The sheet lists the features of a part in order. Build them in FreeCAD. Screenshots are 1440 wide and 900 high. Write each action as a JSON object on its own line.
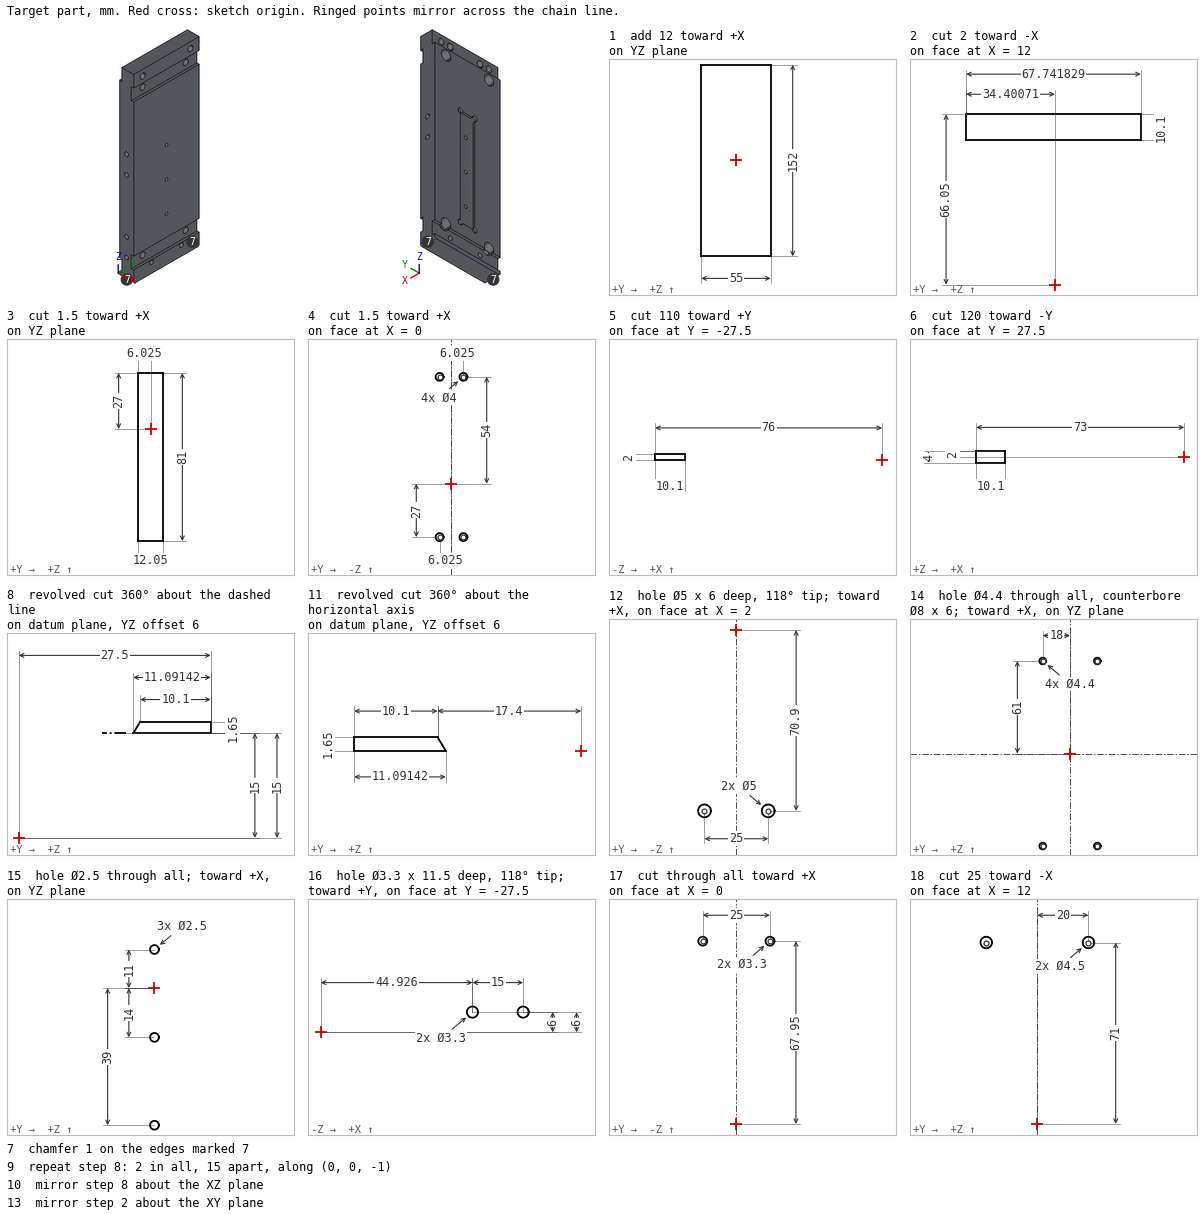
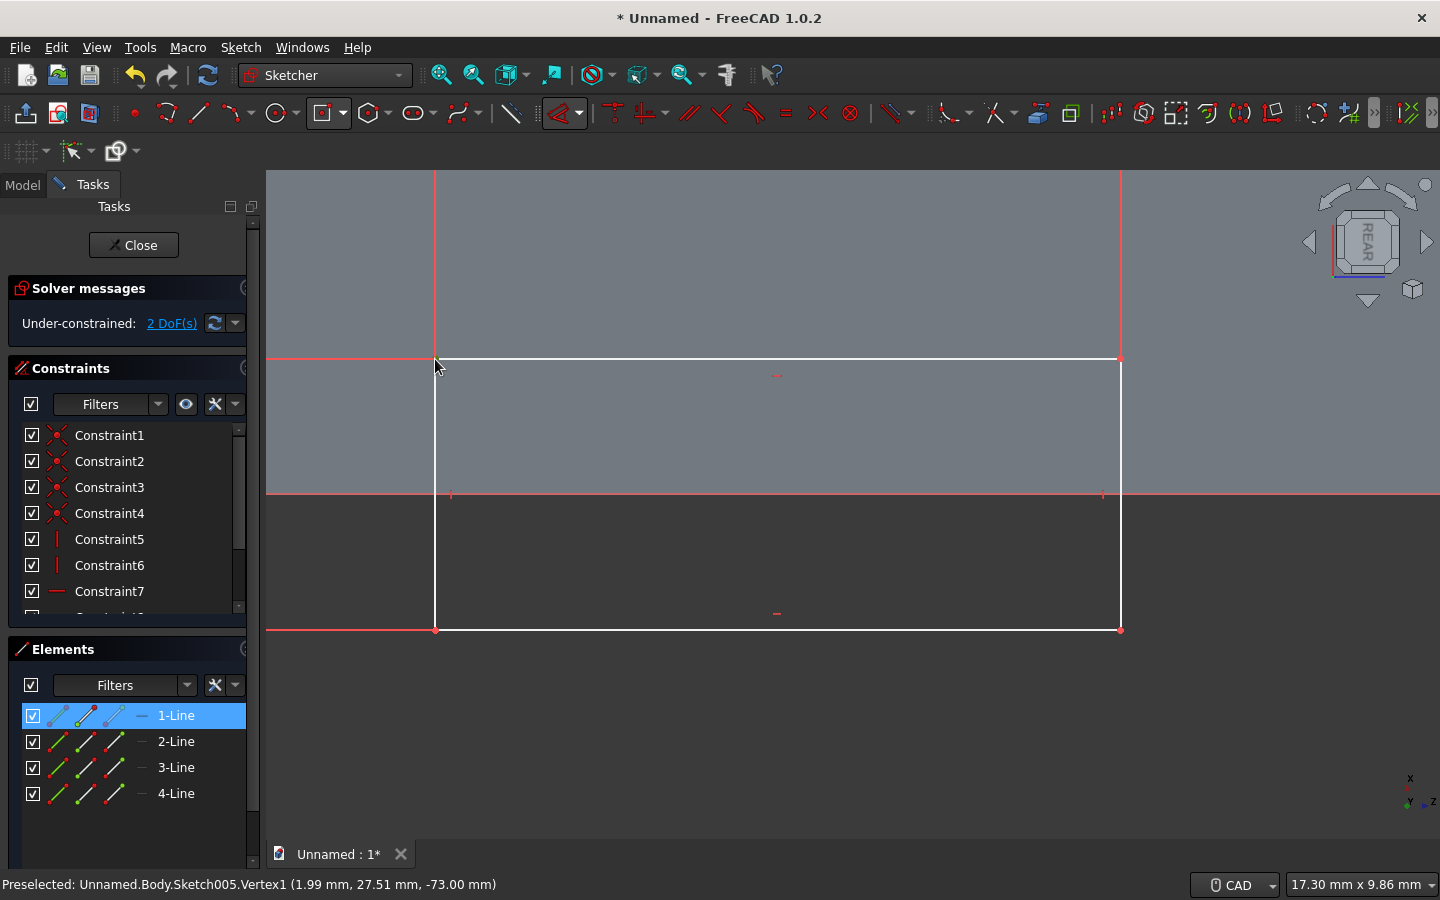
{"action": "left_click", "coordinate": [582, 114]}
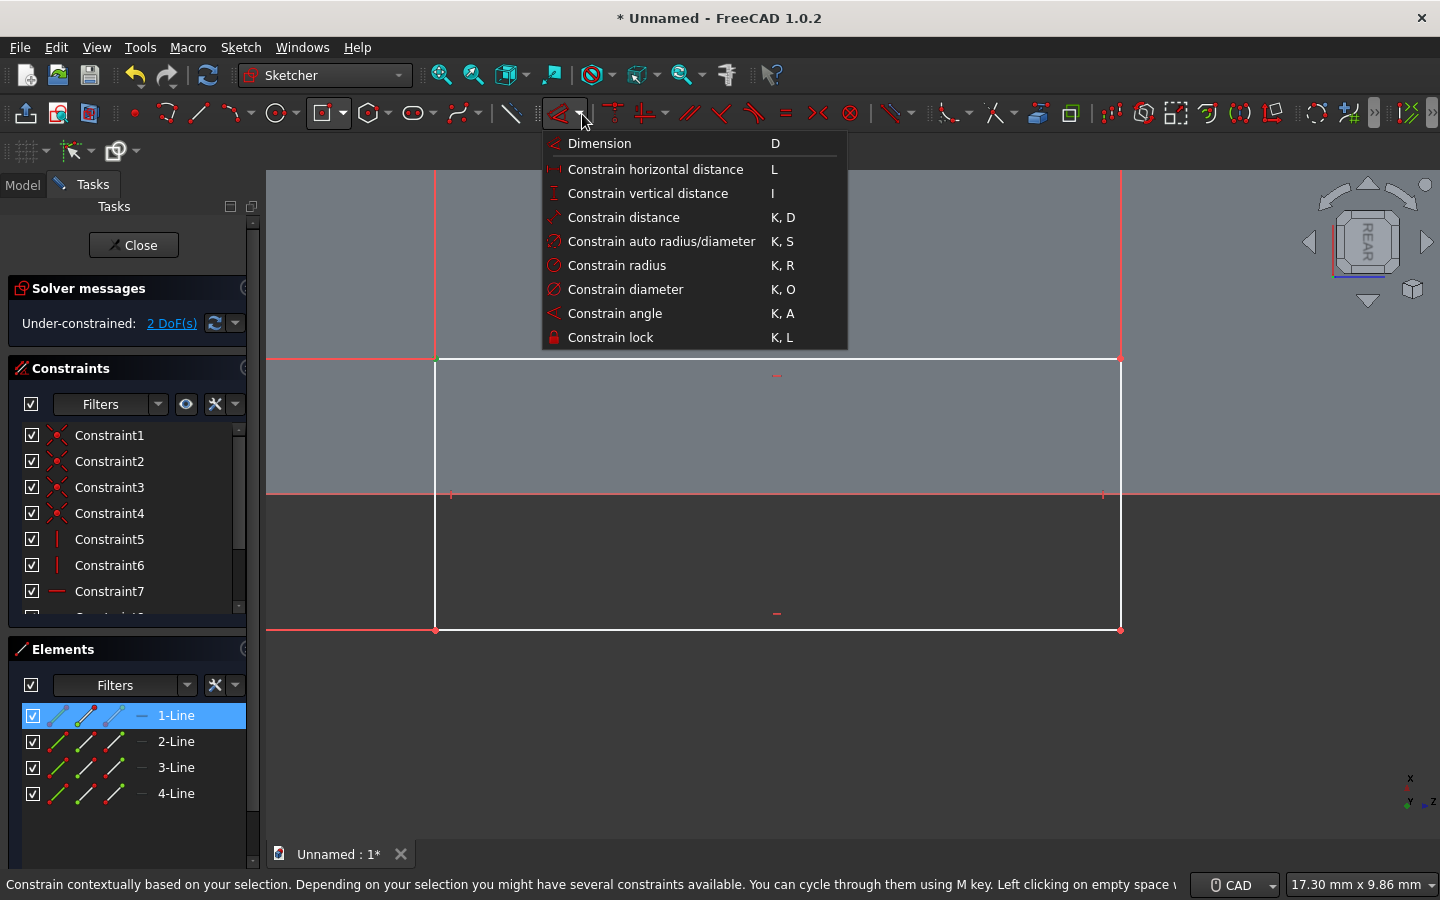
{"action": "left_click", "coordinate": [695, 193]}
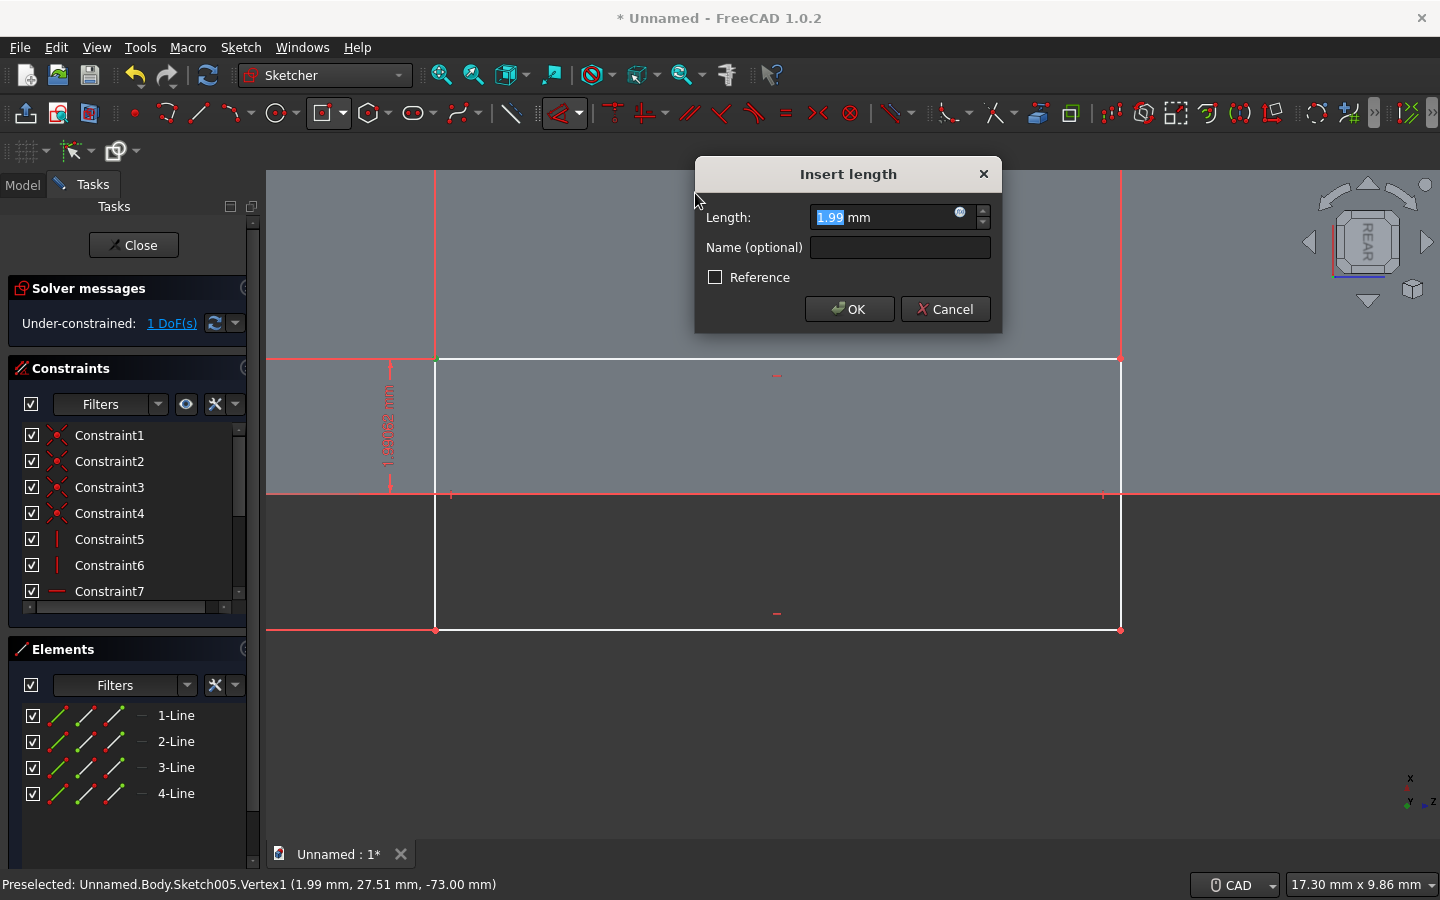
{"action": "type", "text": "2"}
{"action": "key", "text": "Return"}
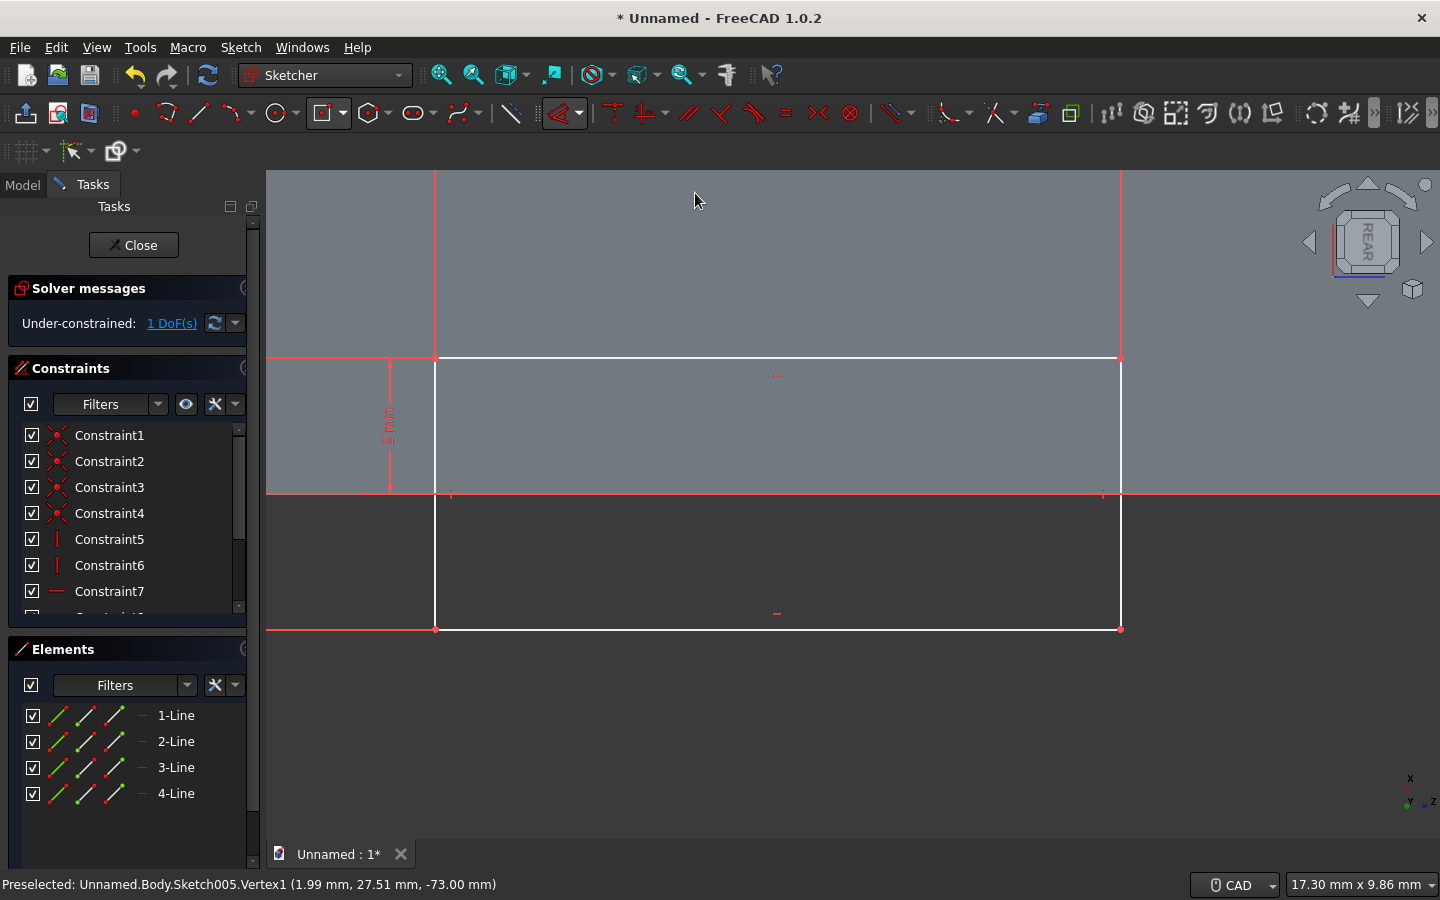
{"action": "left_click", "coordinate": [435, 358]}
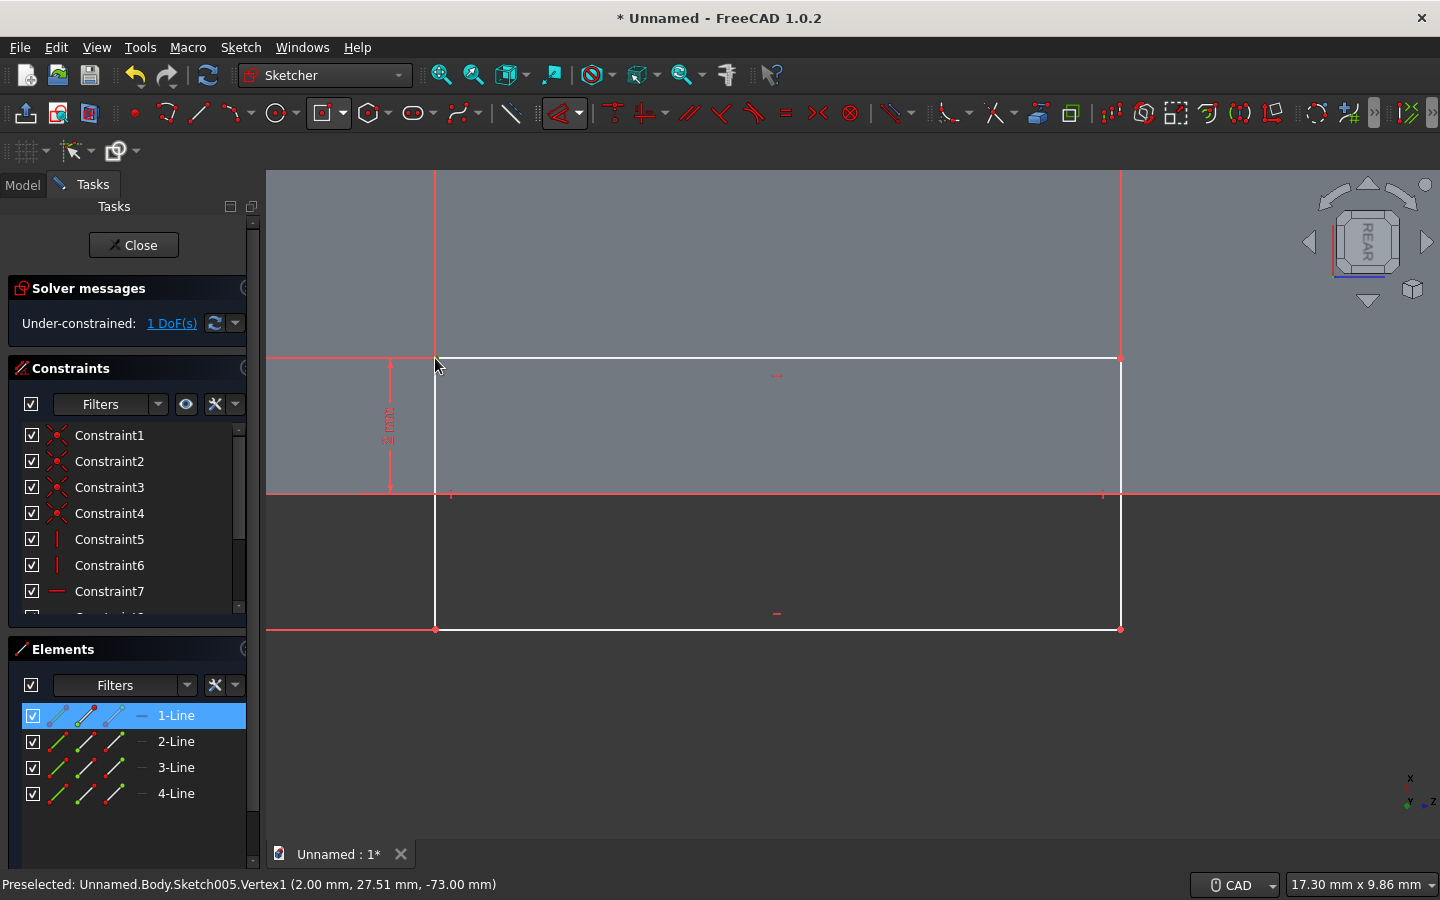
{"action": "left_click", "coordinate": [582, 114]}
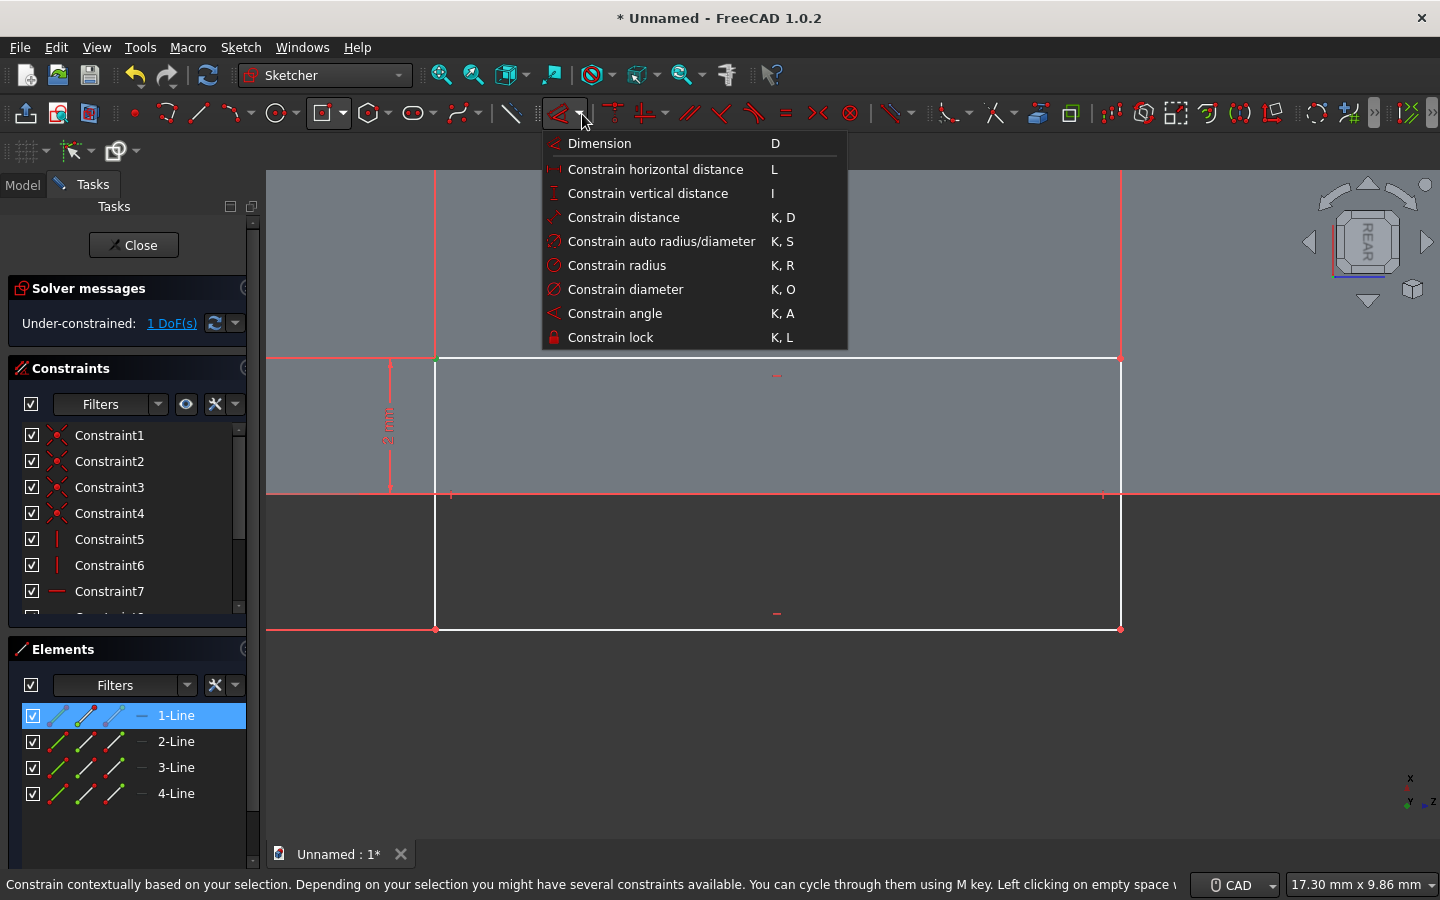
{"action": "left_click", "coordinate": [695, 169]}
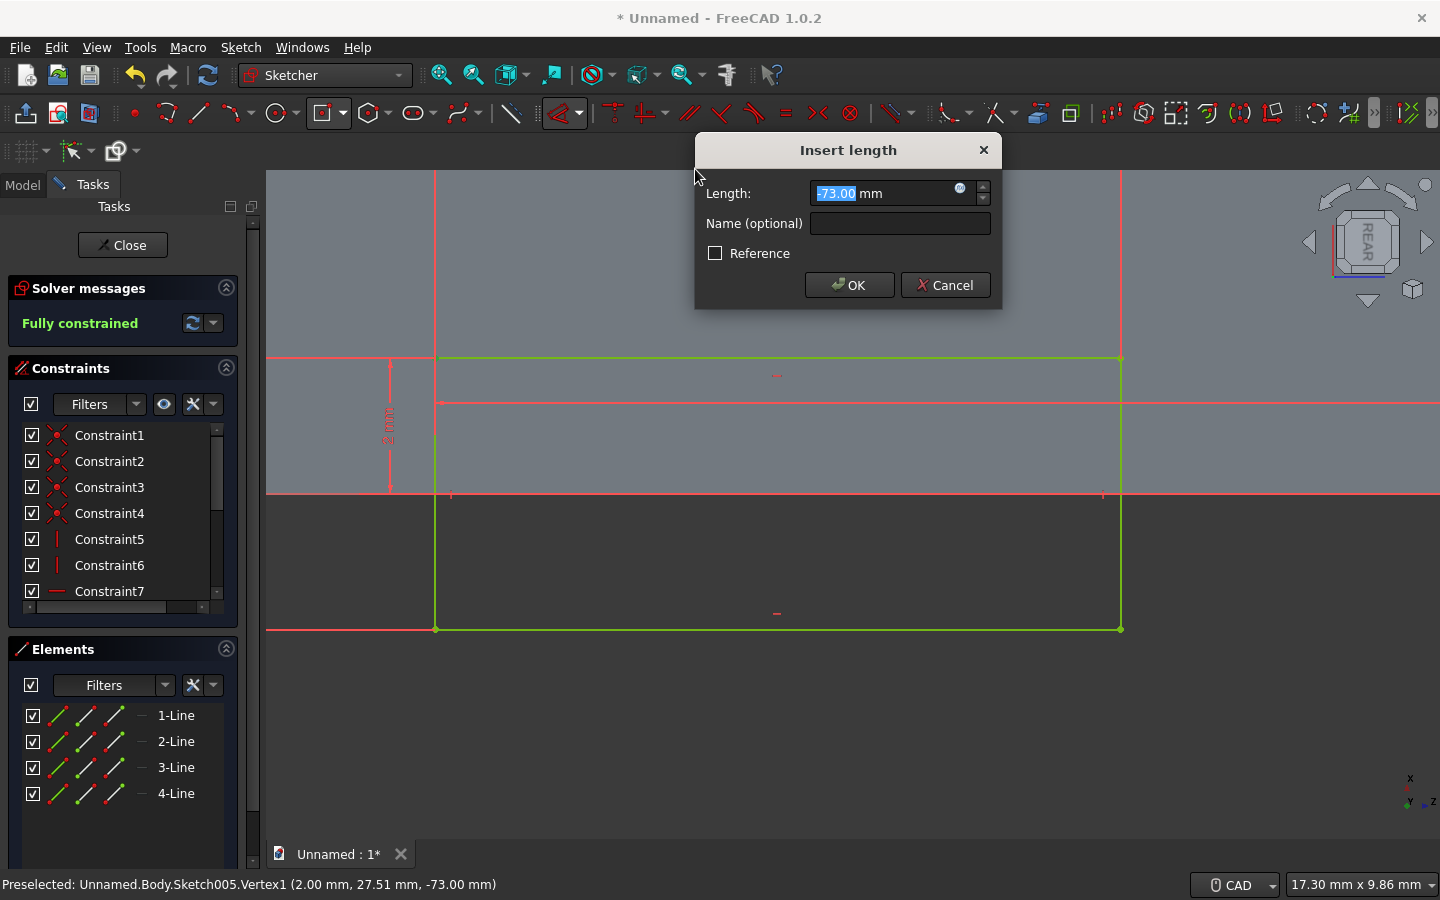
{"action": "type", "text": "-73"}
{"action": "key", "text": "Return"}